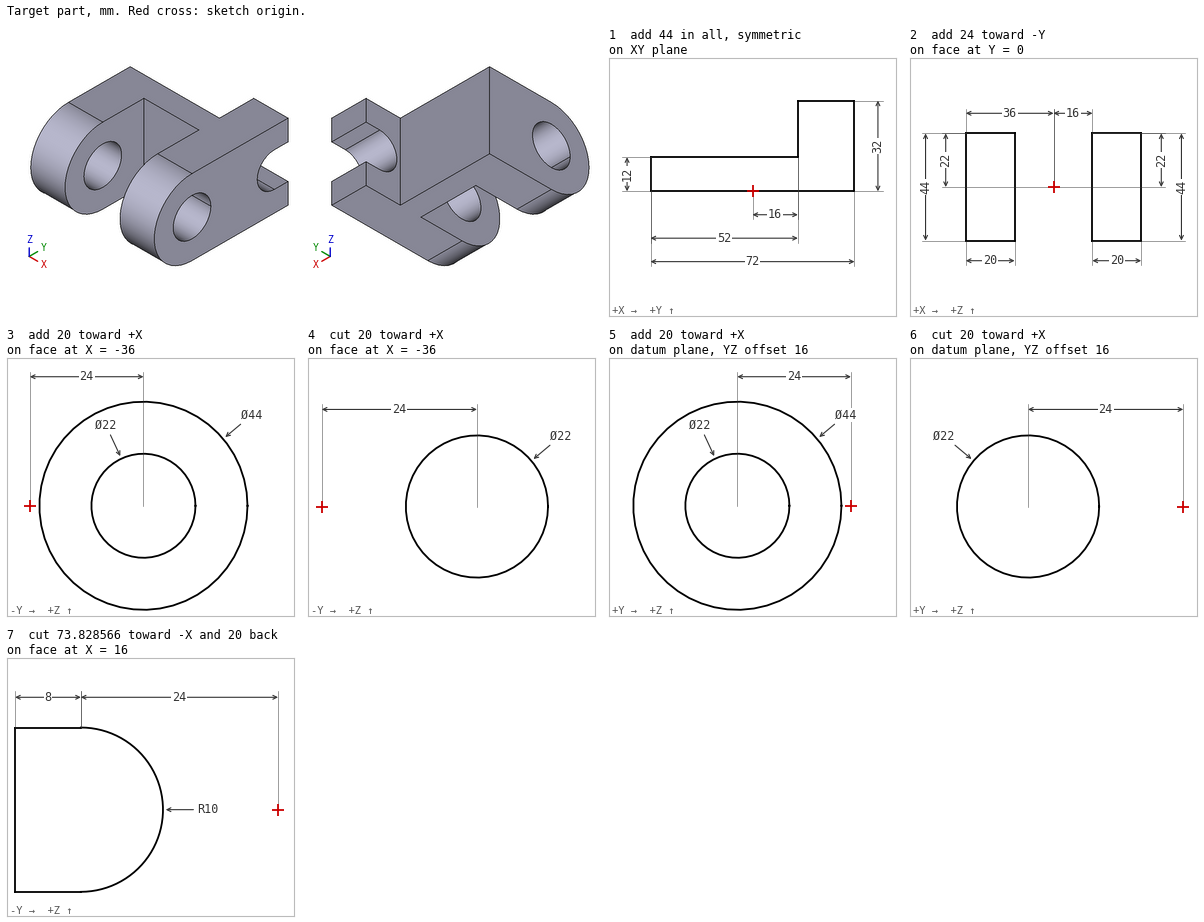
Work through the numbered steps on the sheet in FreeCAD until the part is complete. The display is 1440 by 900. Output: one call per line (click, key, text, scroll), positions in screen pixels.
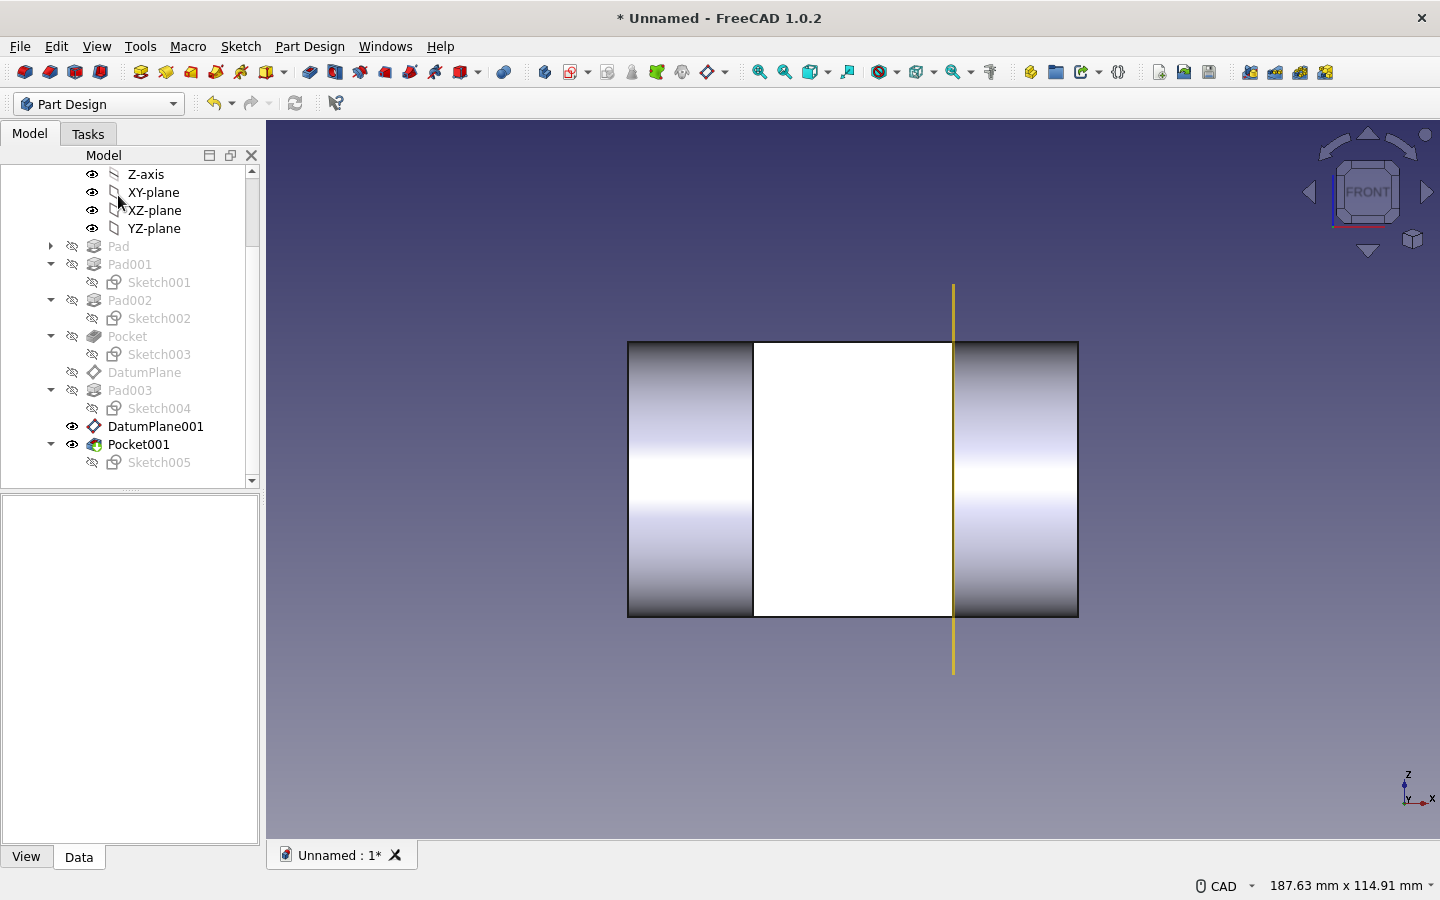
click(117, 426)
key(space)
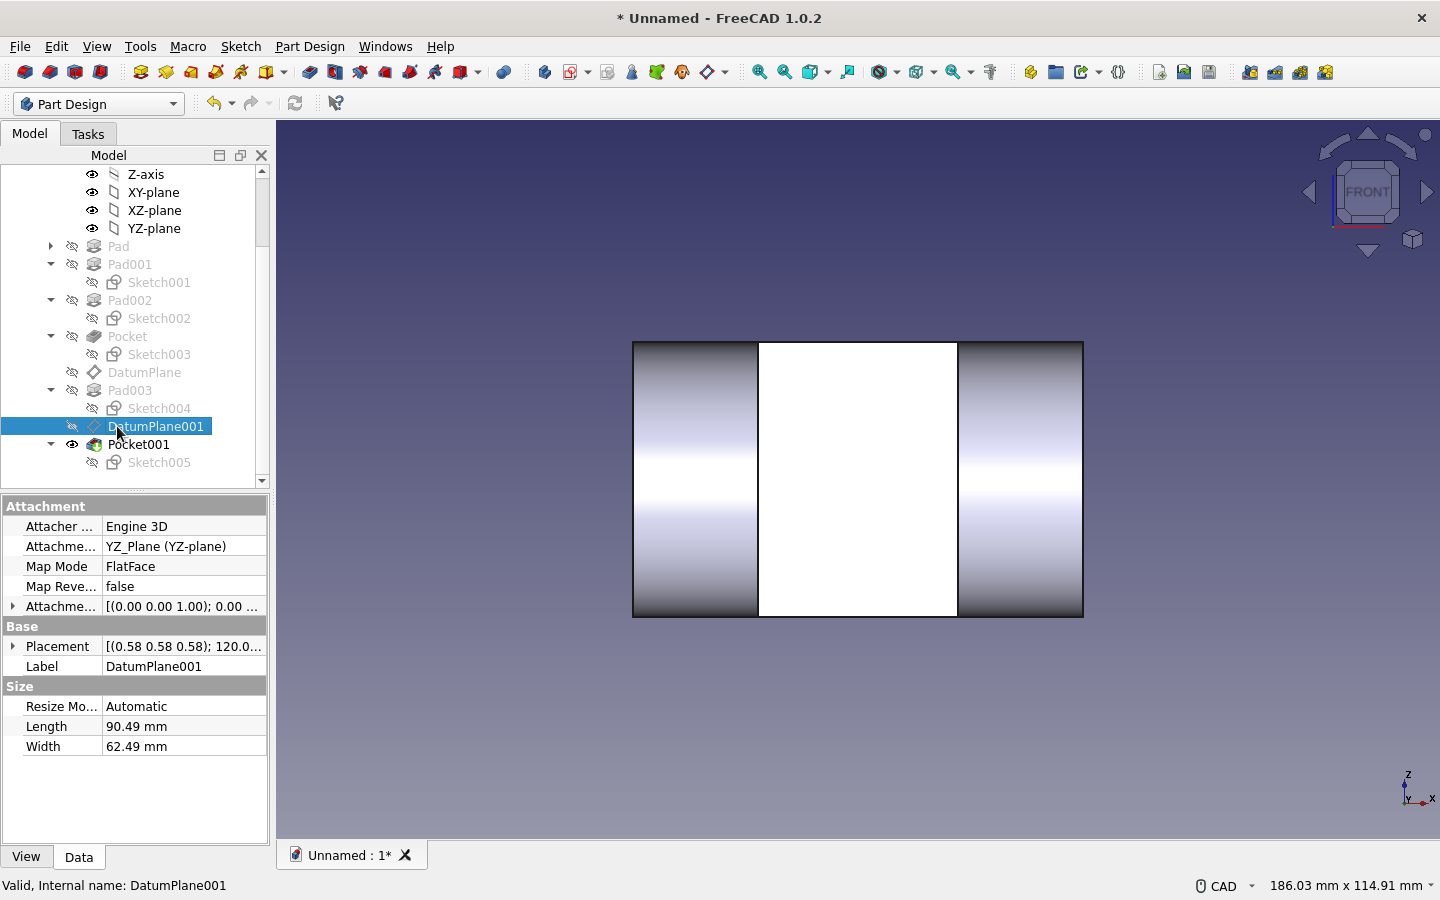
click(760, 72)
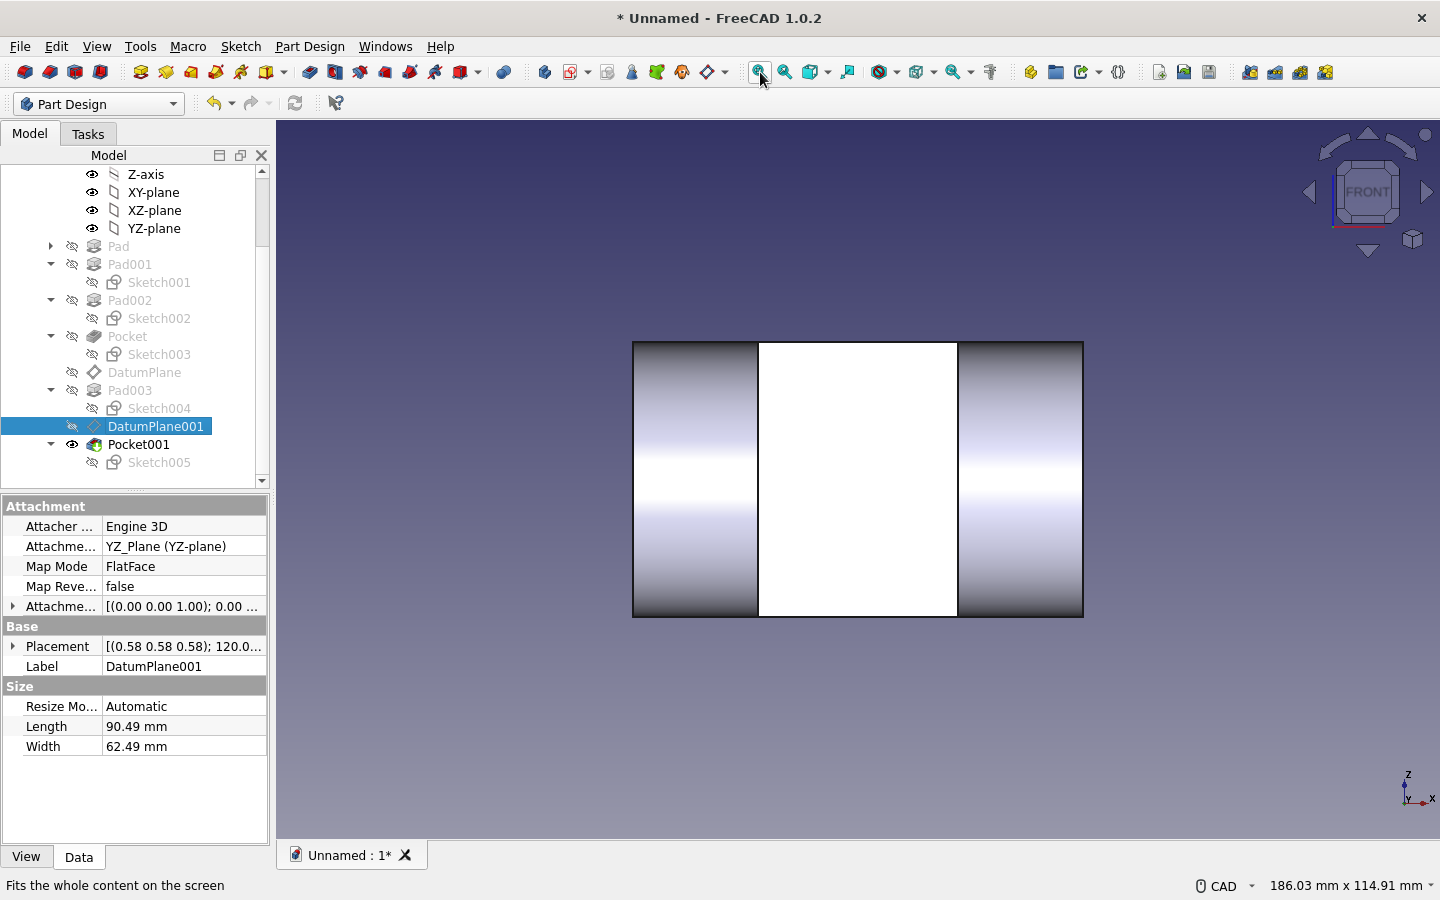
key(6)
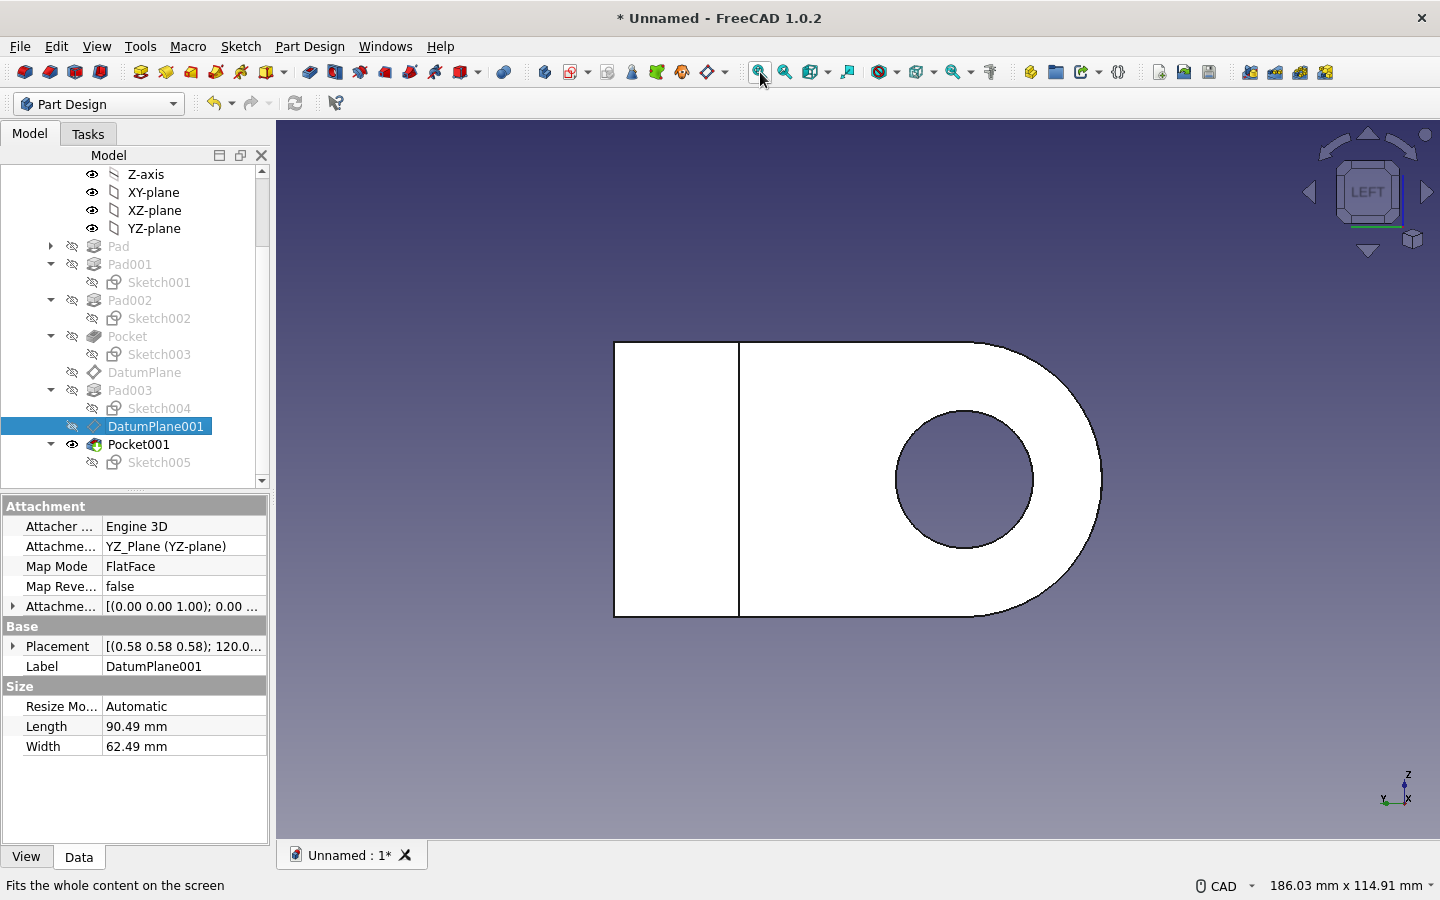
click(760, 72)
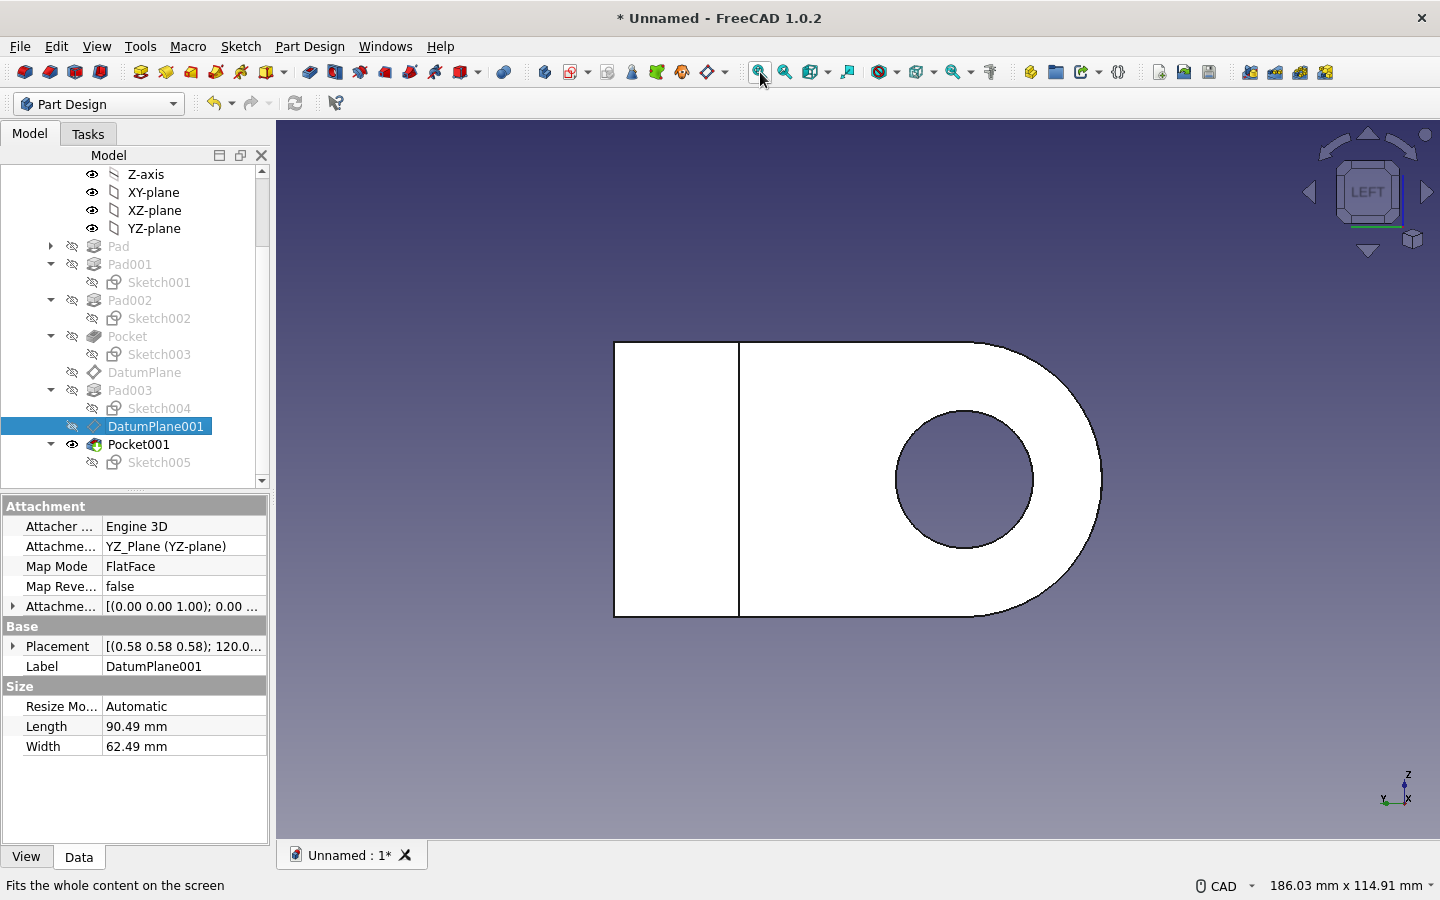
click(677, 439)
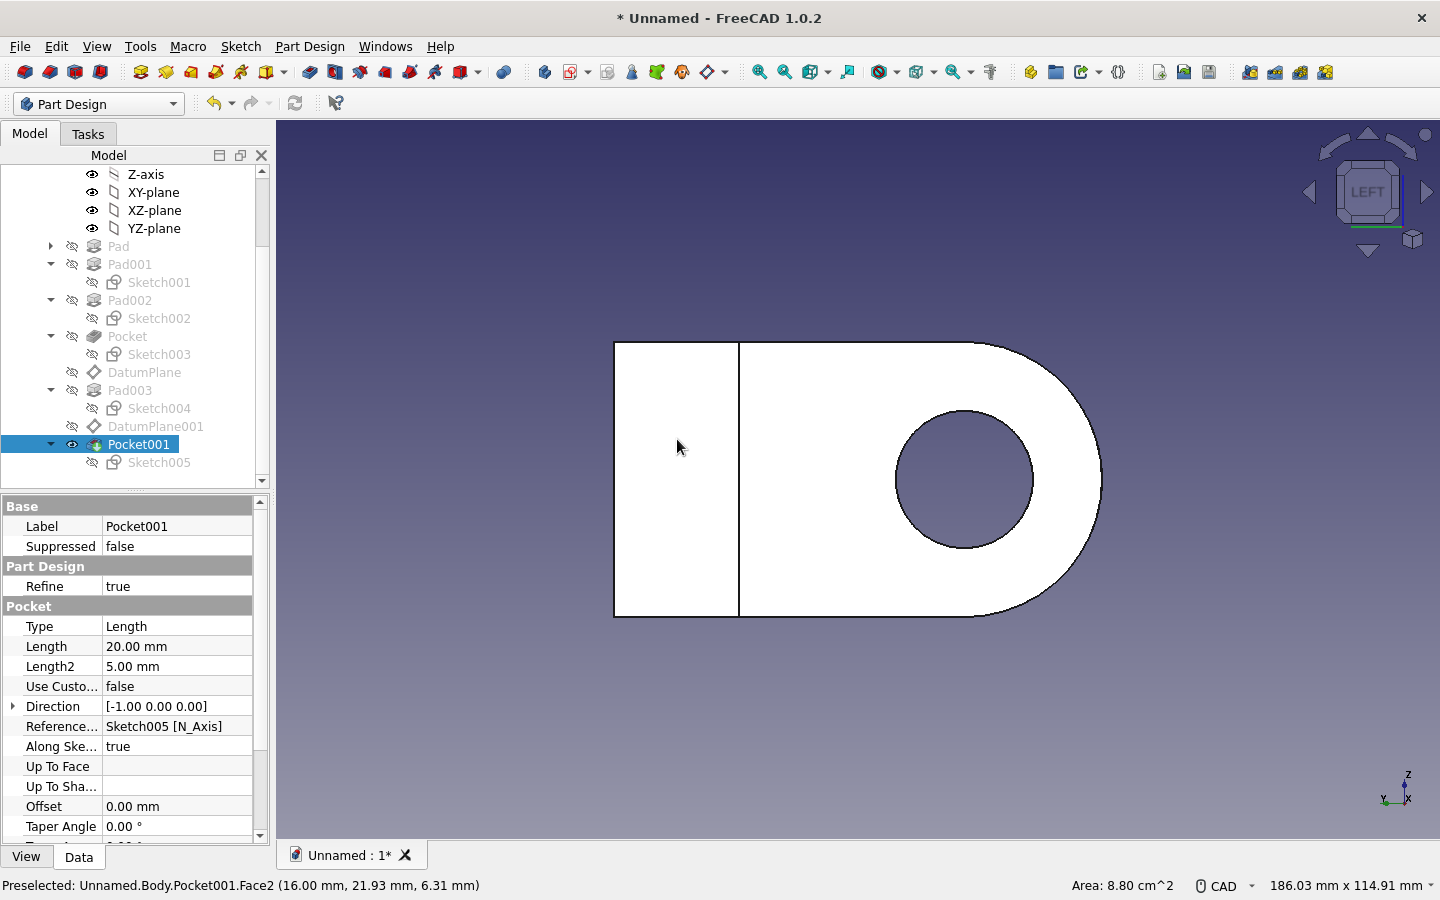
click(570, 72)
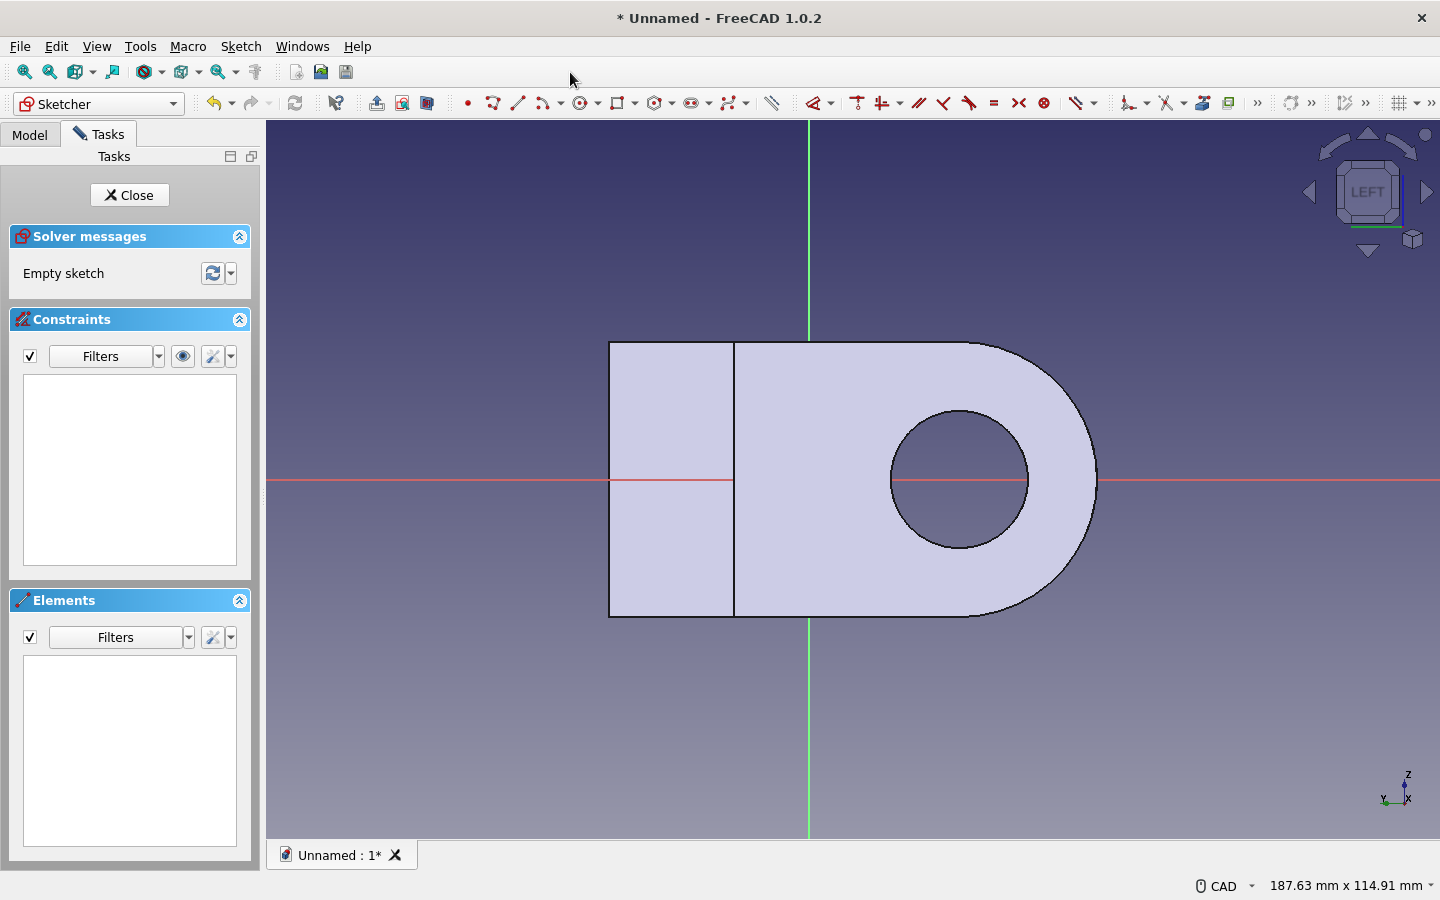
click(427, 104)